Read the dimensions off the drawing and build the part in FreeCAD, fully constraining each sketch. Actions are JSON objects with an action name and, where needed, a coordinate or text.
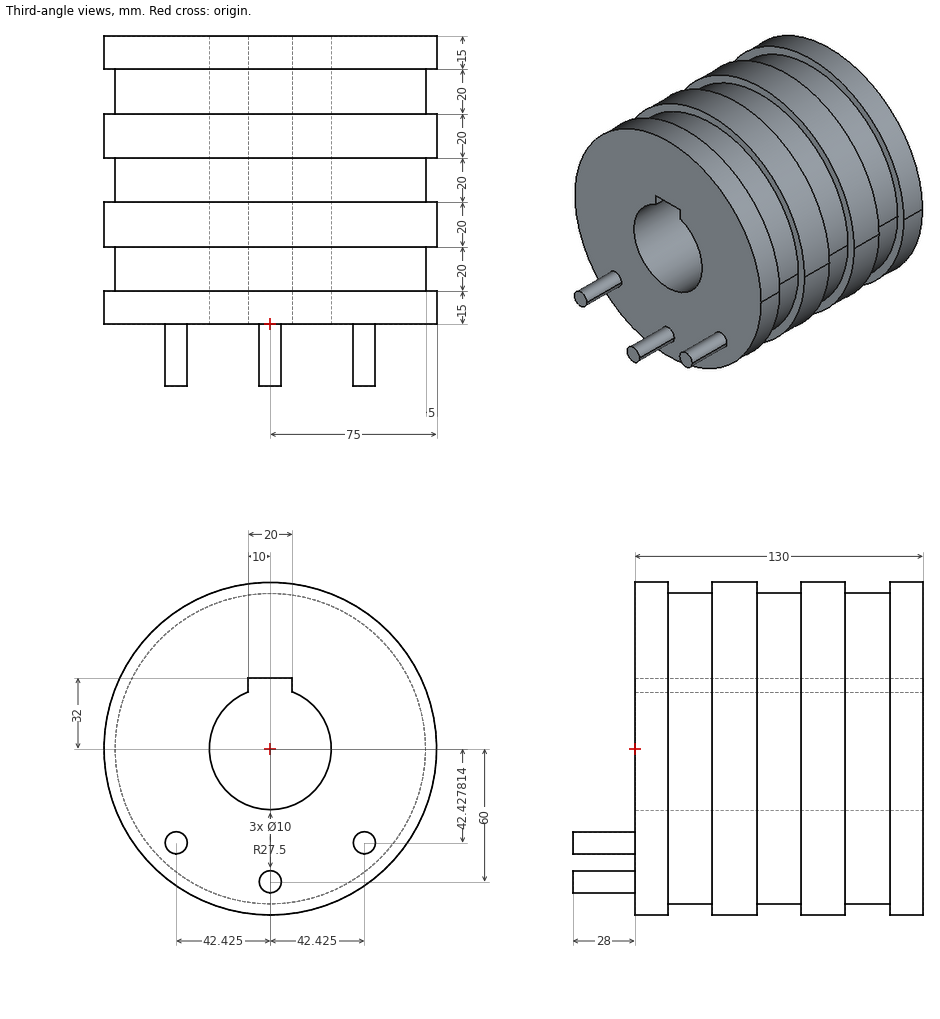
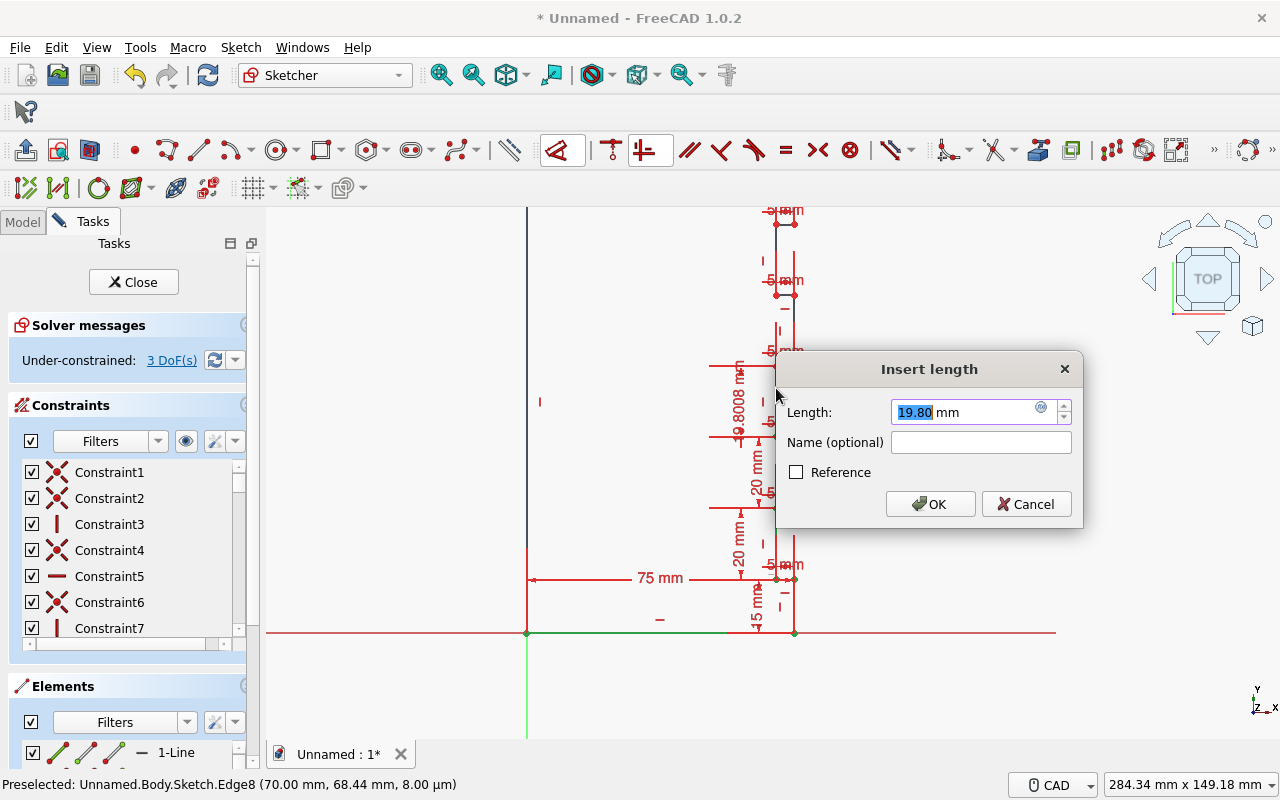
{"action": "type", "text": "20"}
{"action": "key", "text": "Return"}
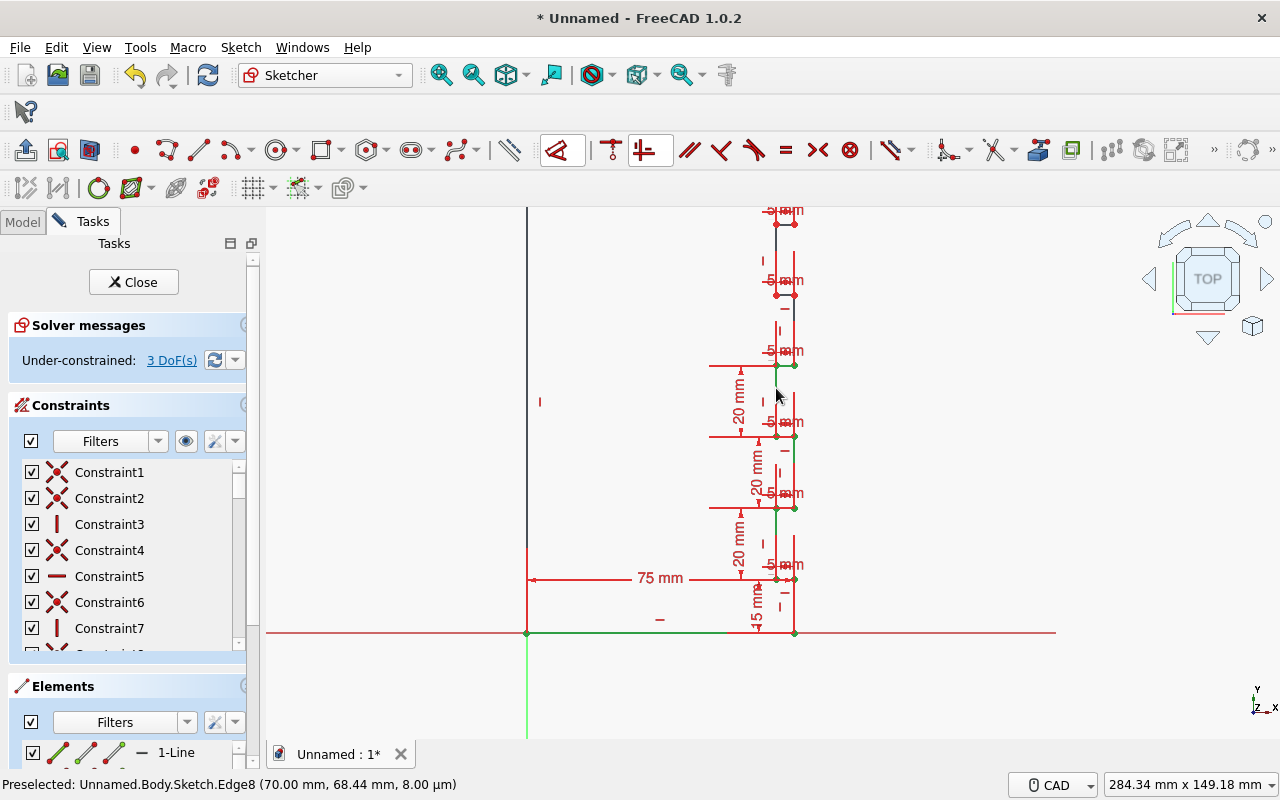
{"action": "left_click", "coordinate": [794, 316]}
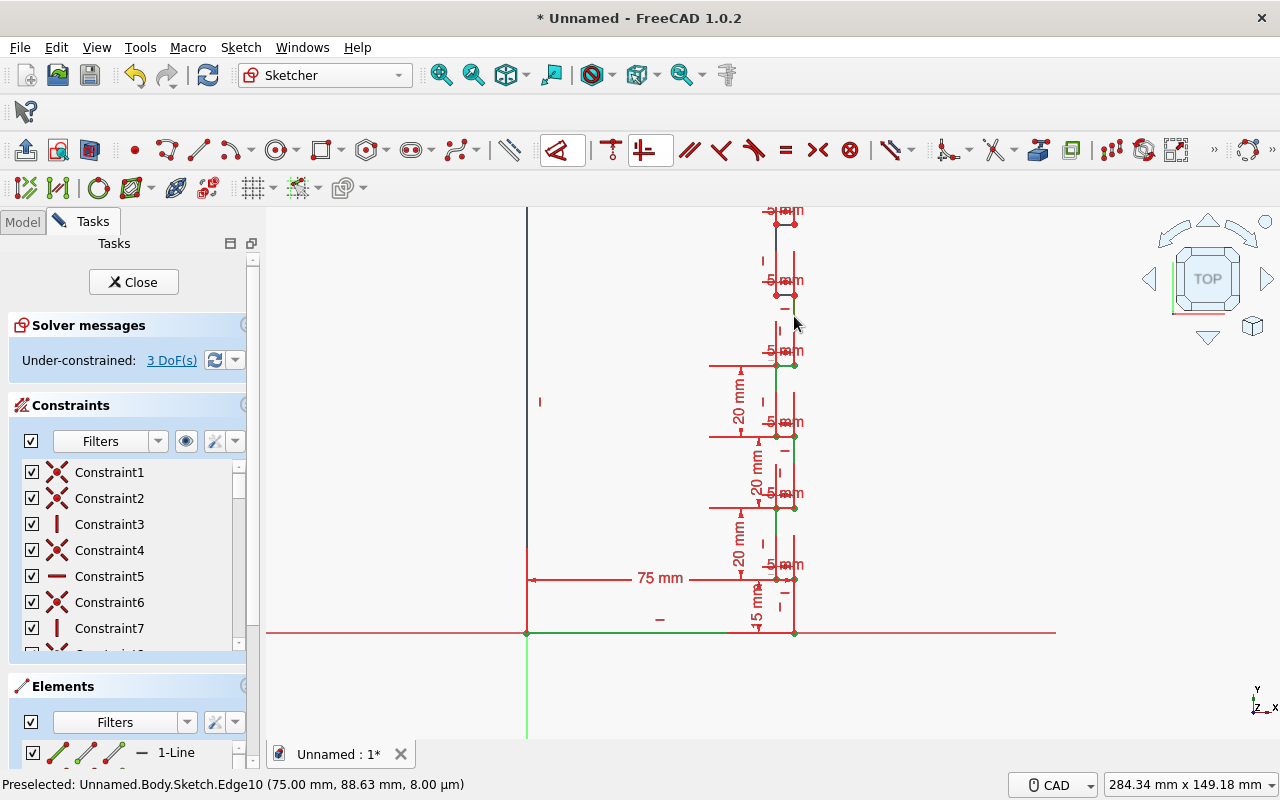
{"action": "key", "text": "i"}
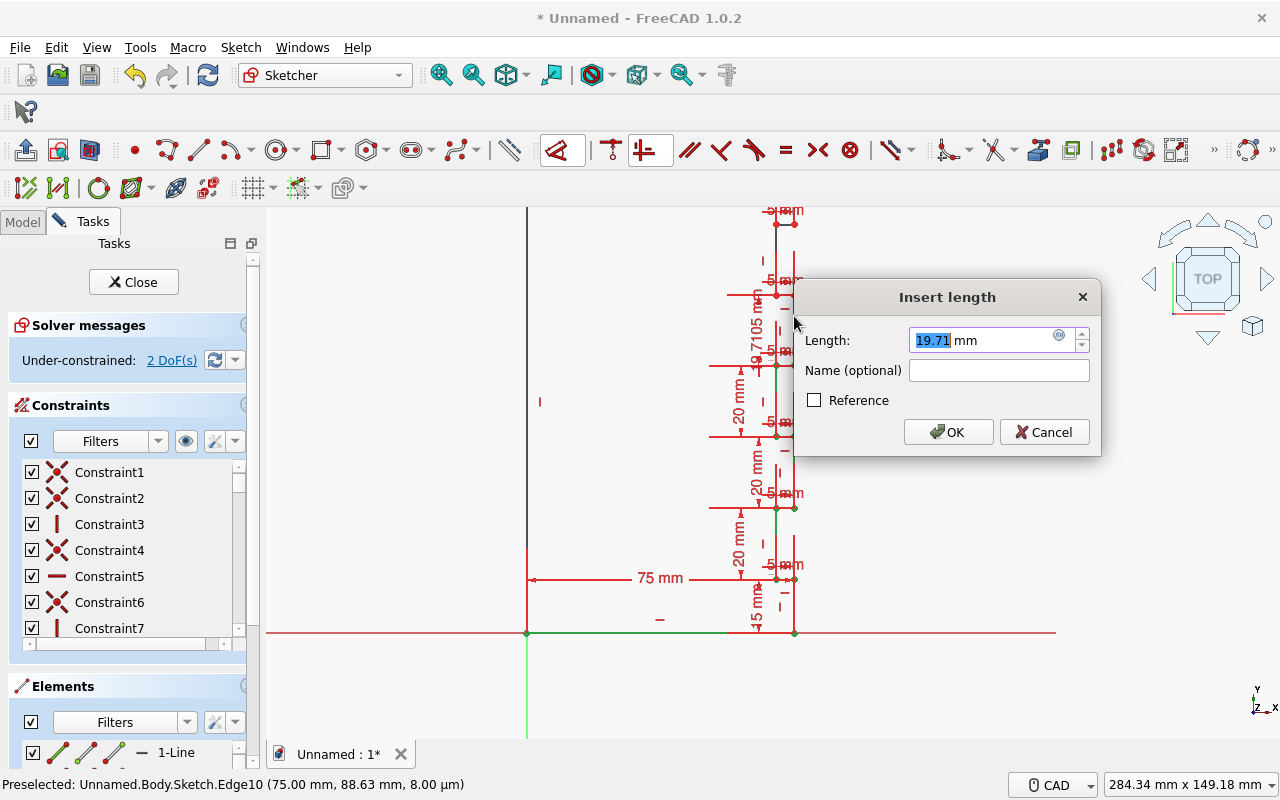
{"action": "type", "text": "20"}
{"action": "key", "text": "Return"}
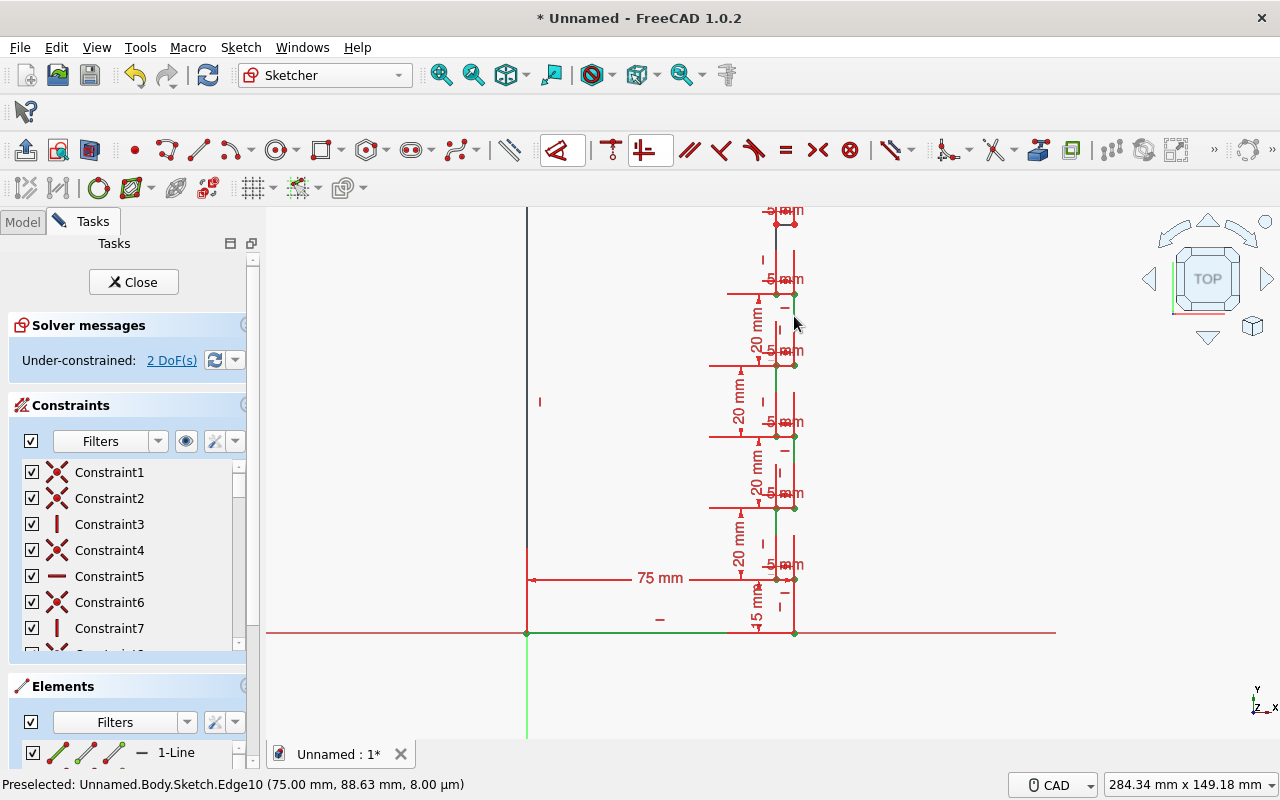
{"action": "left_click", "coordinate": [776, 246]}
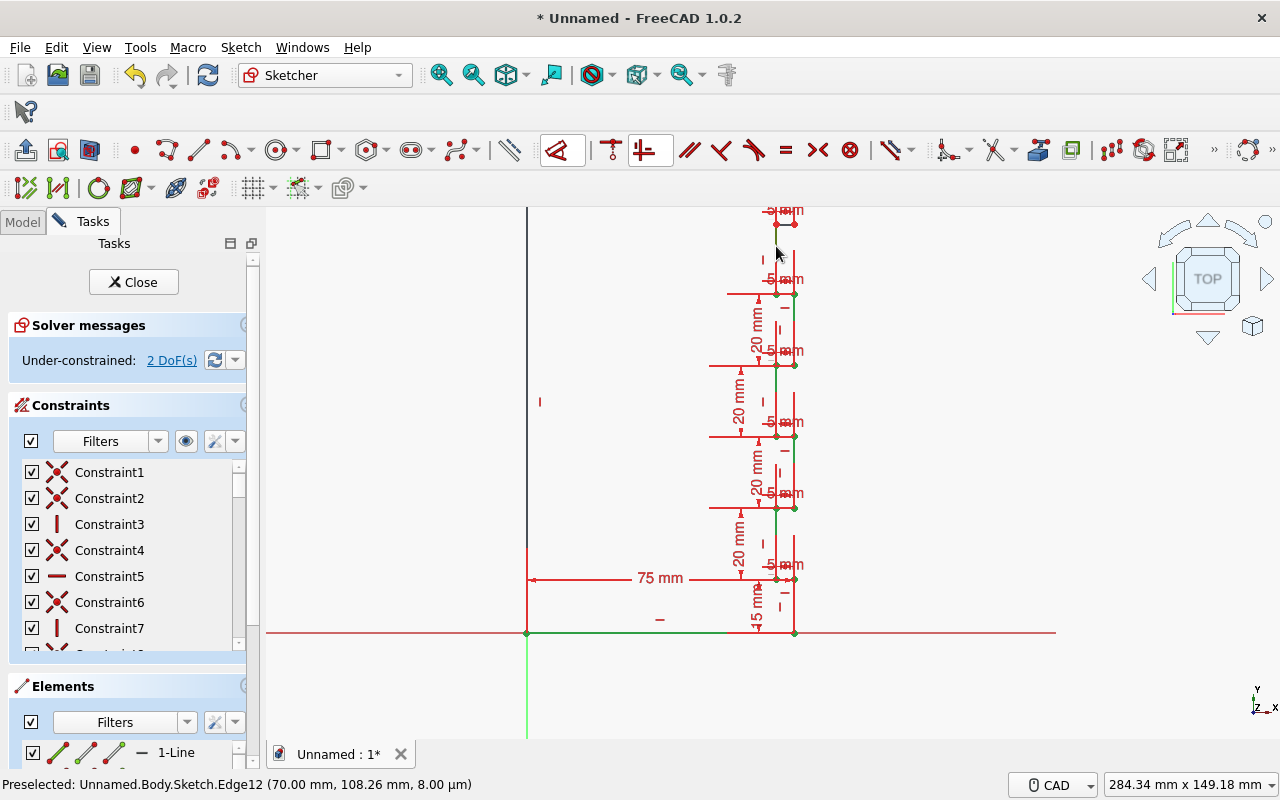
{"action": "key", "text": "i"}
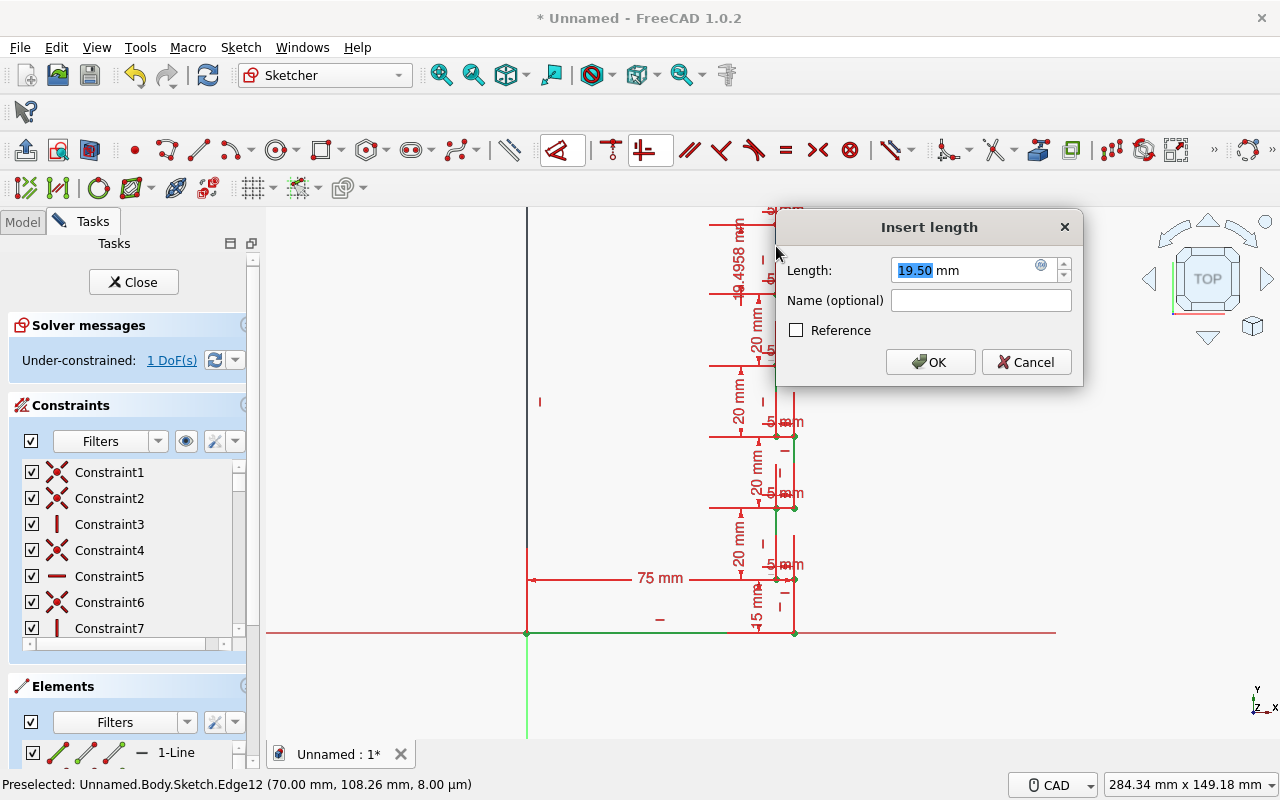
{"action": "type", "text": "20"}
{"action": "key", "text": "Return"}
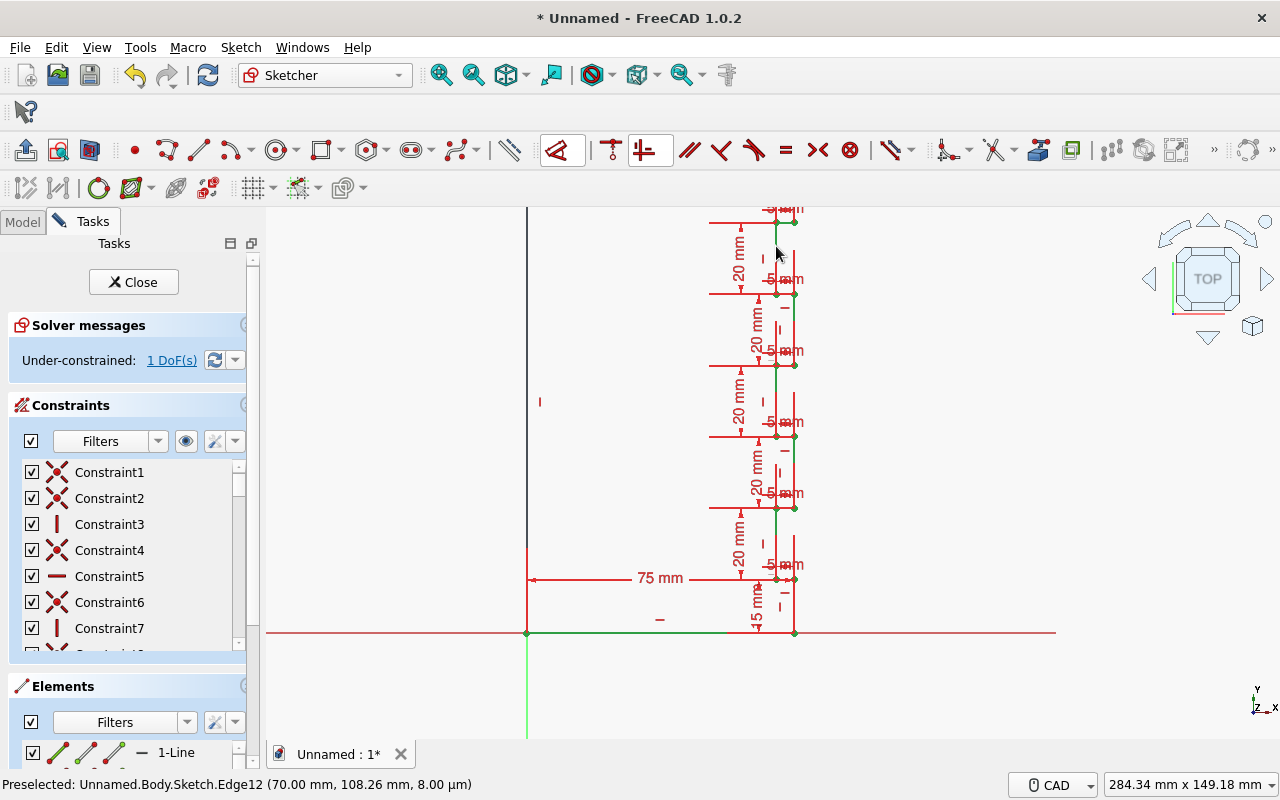
{"action": "scroll", "coordinate": [794, 619], "scroll_direction": "down", "scroll_amount": 2}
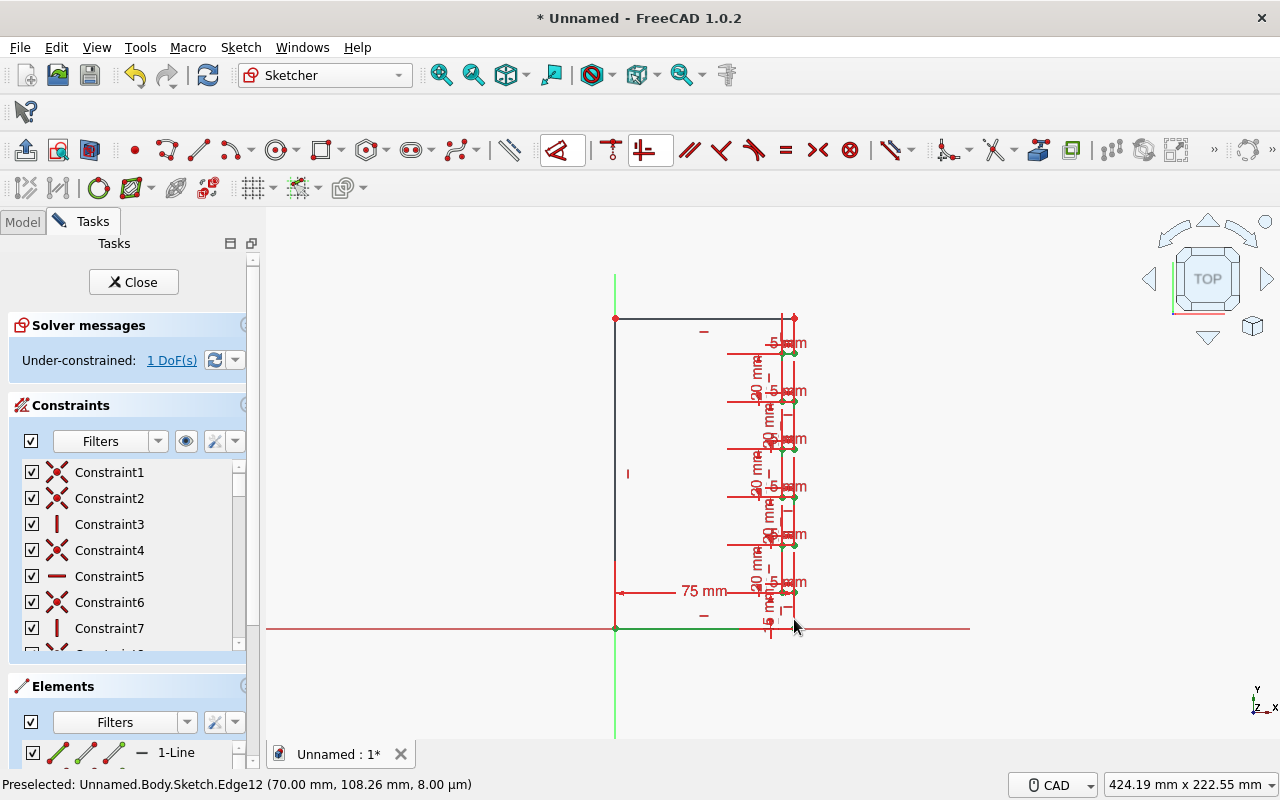
{"action": "scroll", "coordinate": [794, 343], "scroll_direction": "up", "scroll_amount": 2}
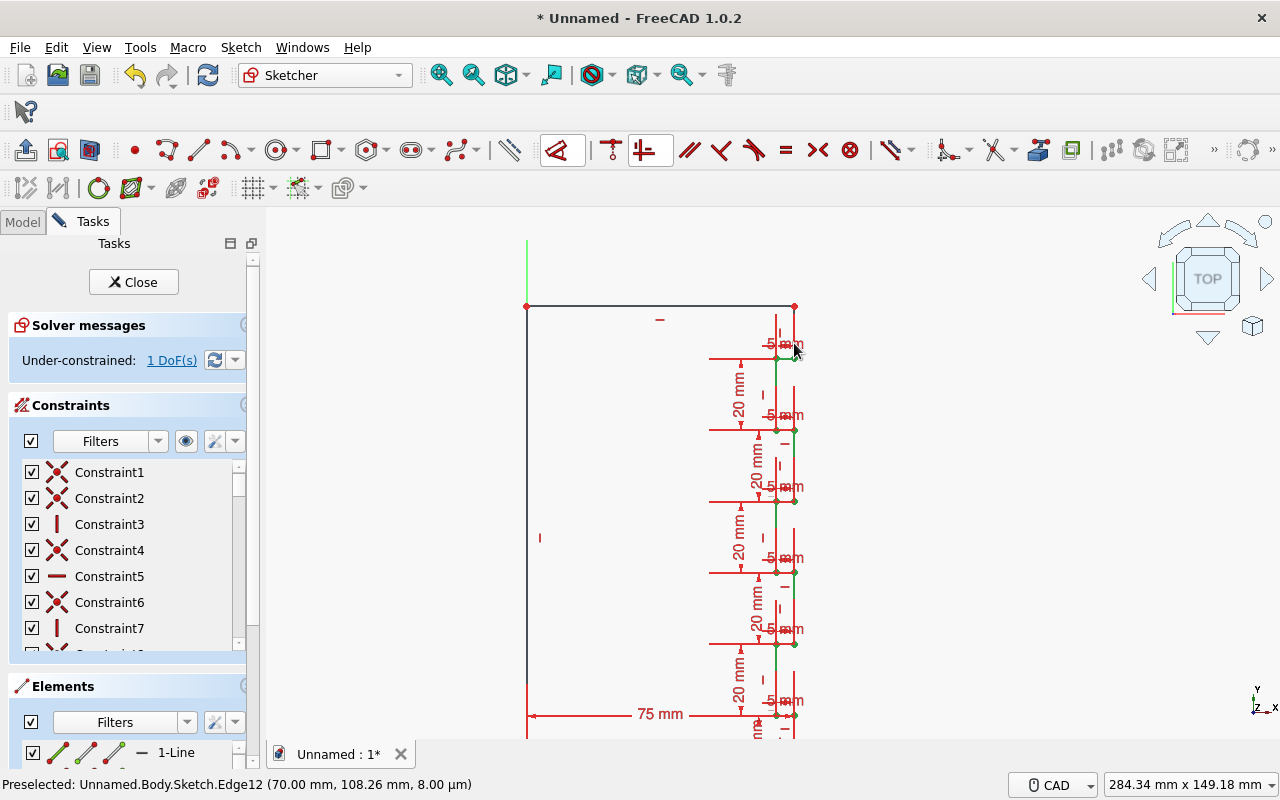
{"action": "left_click", "coordinate": [794, 322]}